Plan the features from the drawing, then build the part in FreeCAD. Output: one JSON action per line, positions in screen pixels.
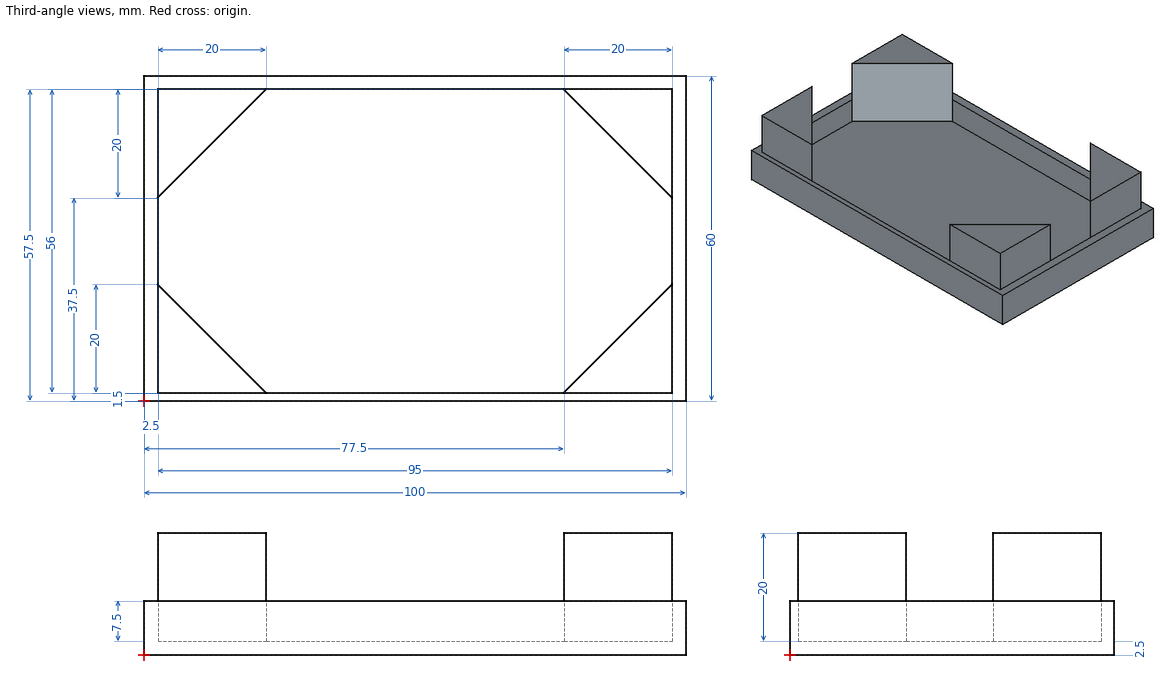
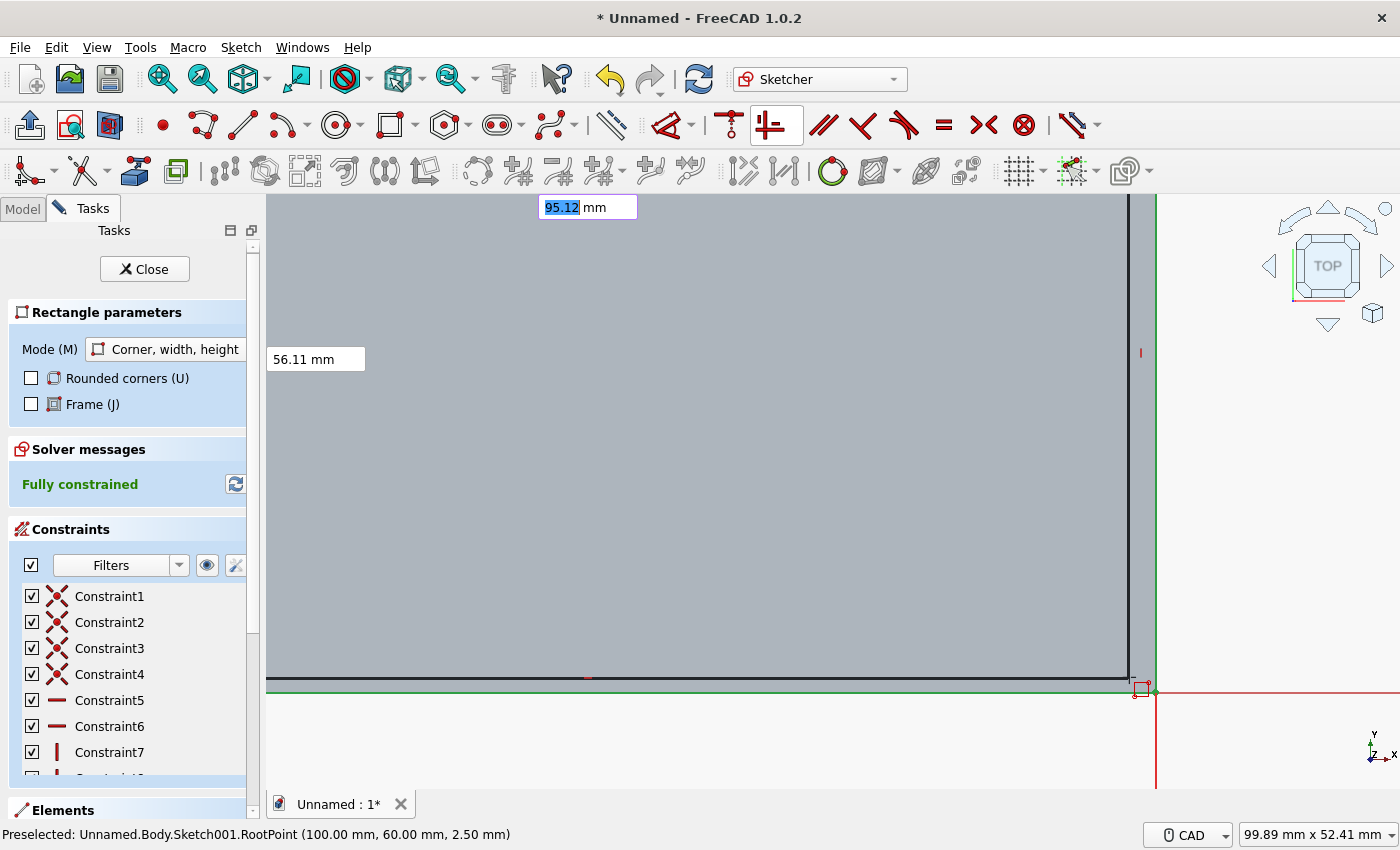
{"action": "left_click", "coordinate": [1128, 676]}
{"action": "key", "text": "Escape"}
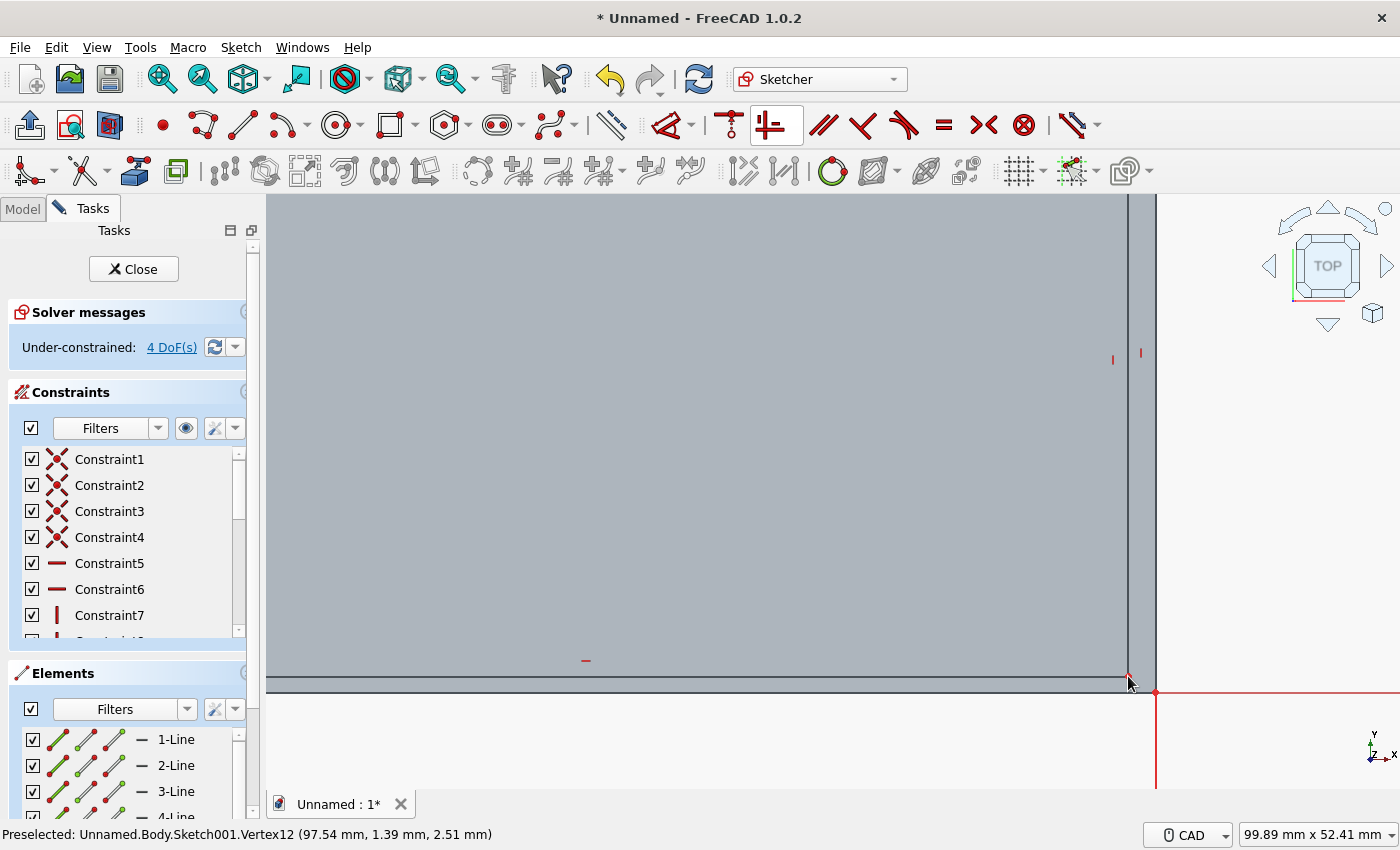
{"action": "left_click", "coordinate": [666, 126]}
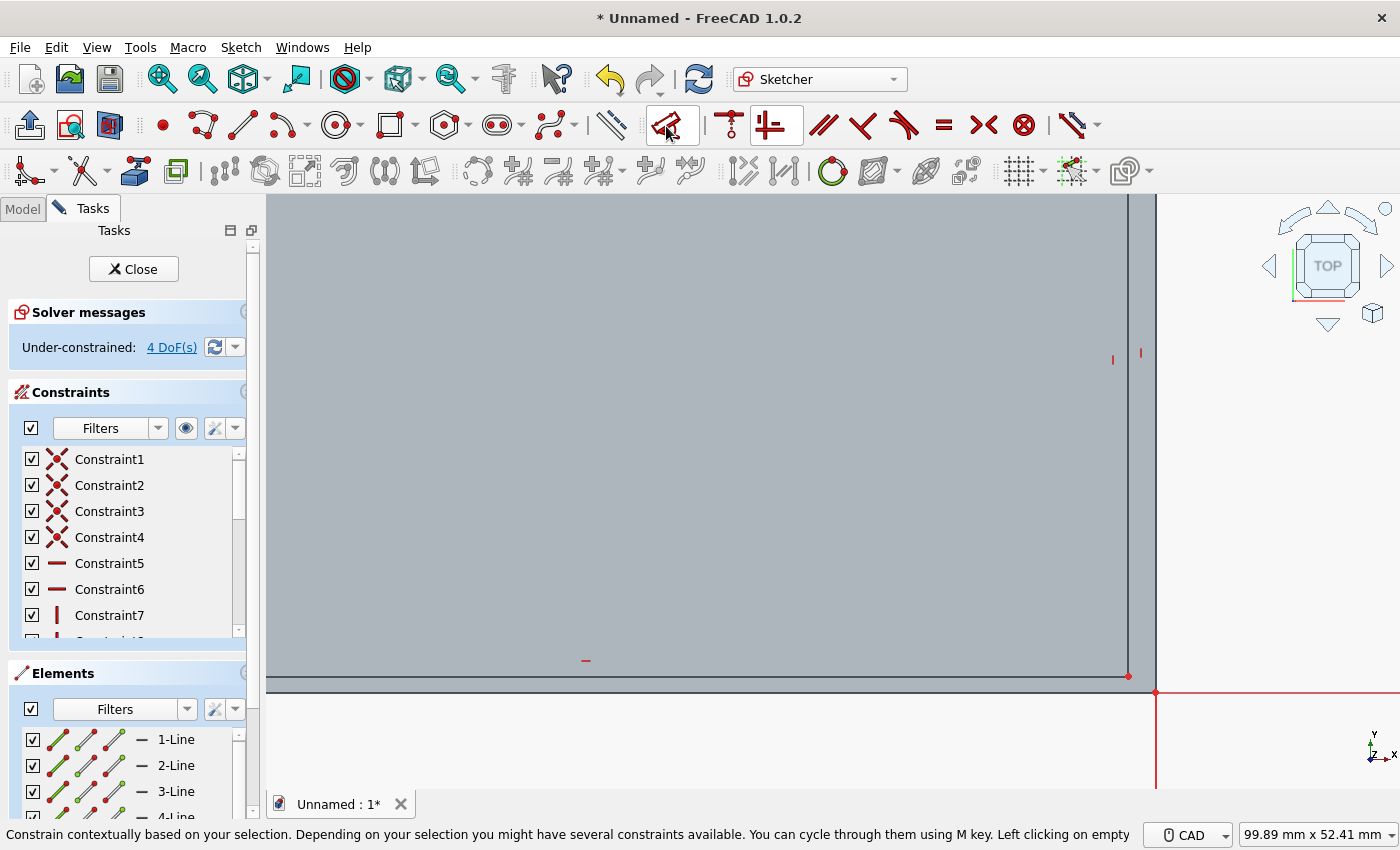
{"action": "scroll", "coordinate": [979, 661], "scroll_direction": "down", "scroll_amount": 3}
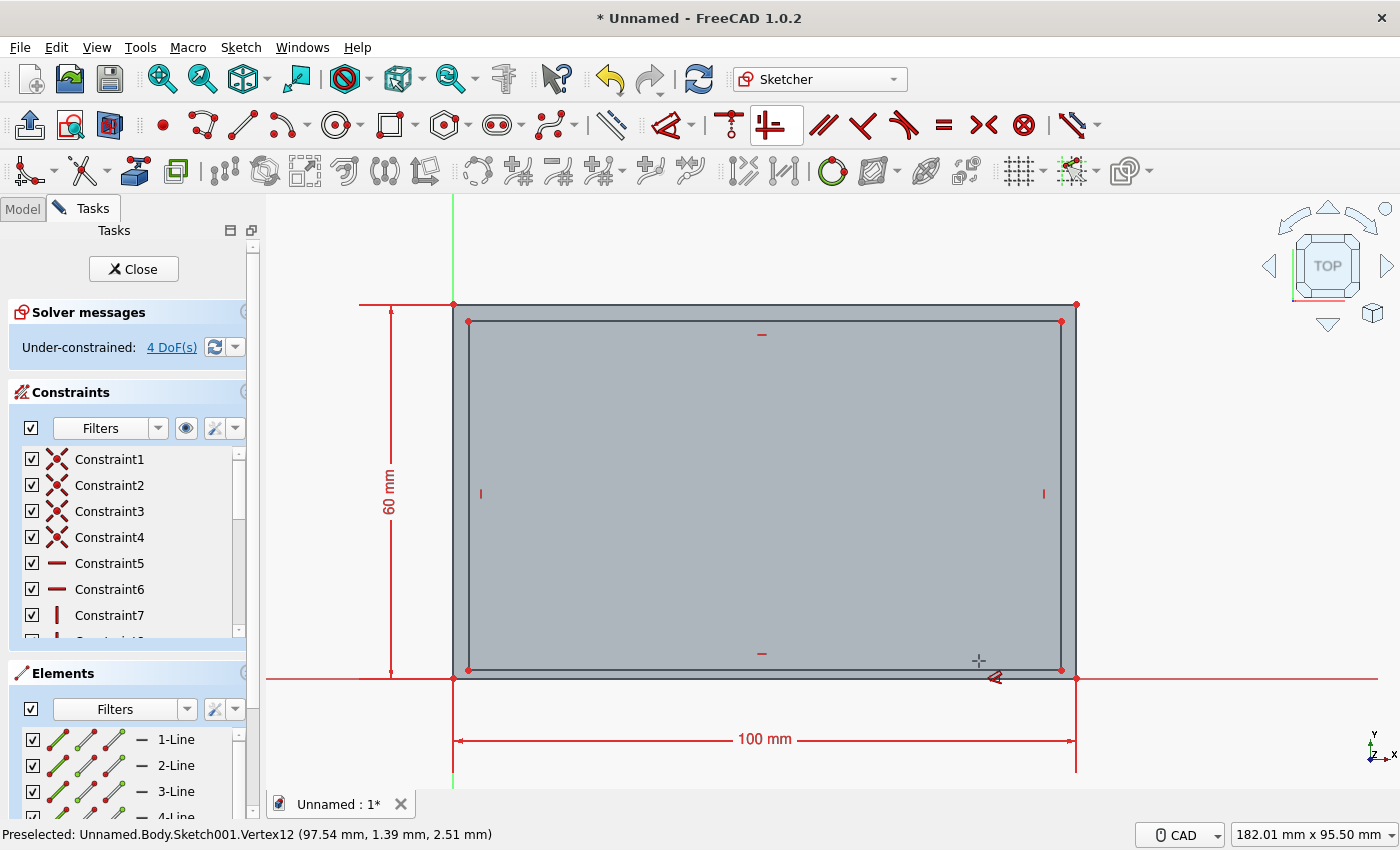
{"action": "left_click", "coordinate": [469, 426]}
{"action": "left_click", "coordinate": [435, 496]}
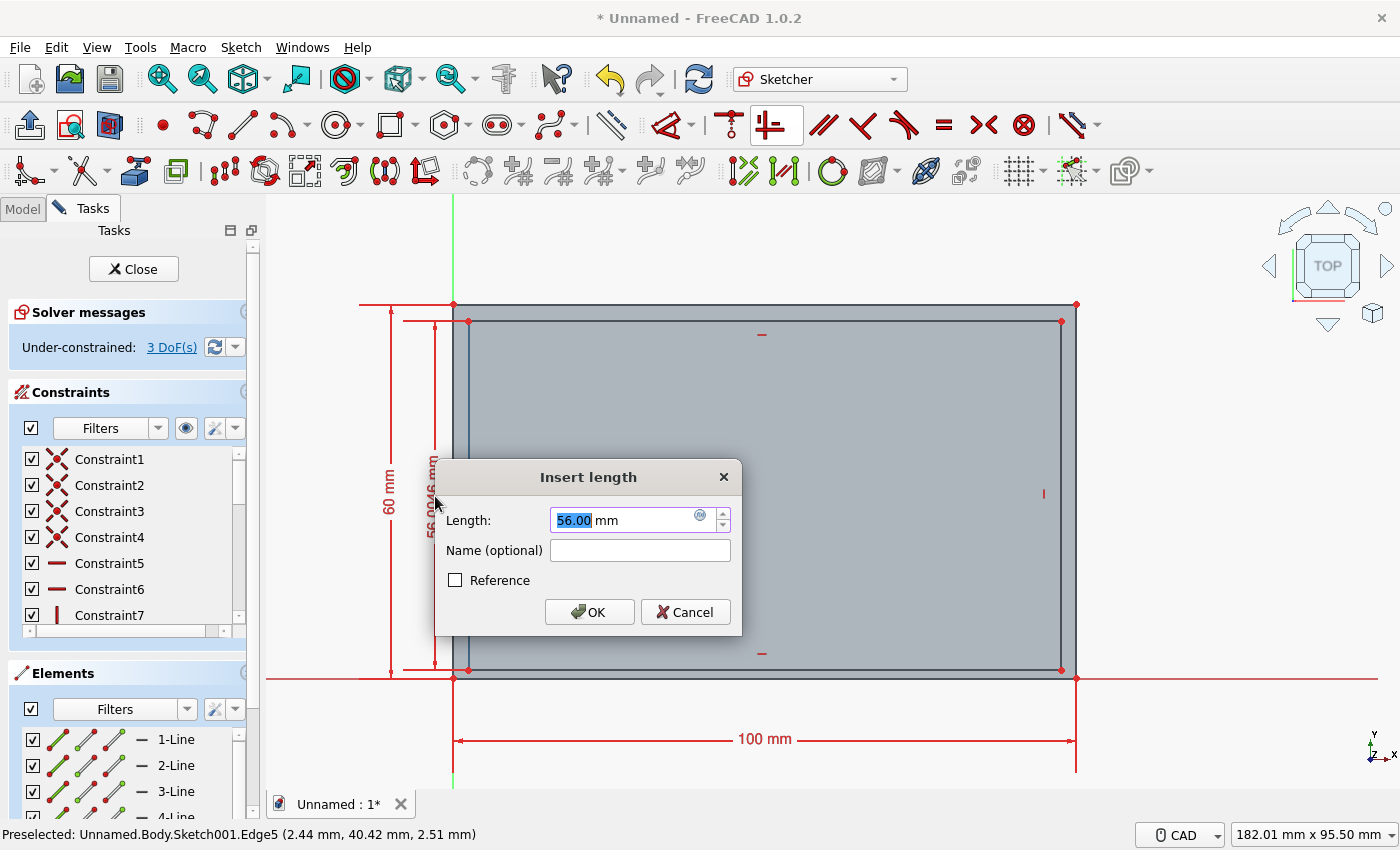
{"action": "type", "text": "56"}
{"action": "key", "text": "Return"}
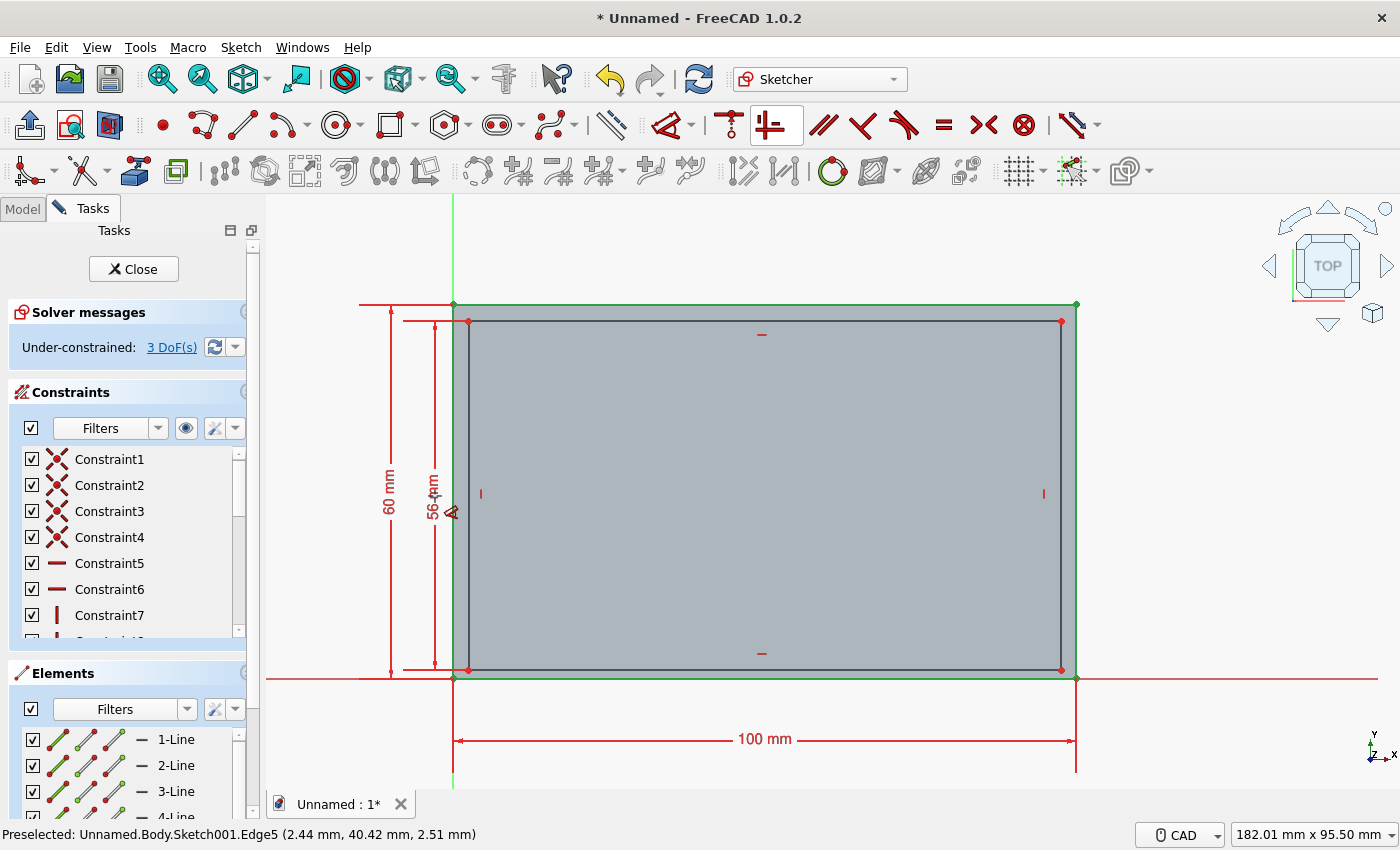
{"action": "scroll", "coordinate": [646, 670], "scroll_direction": "up", "scroll_amount": 3}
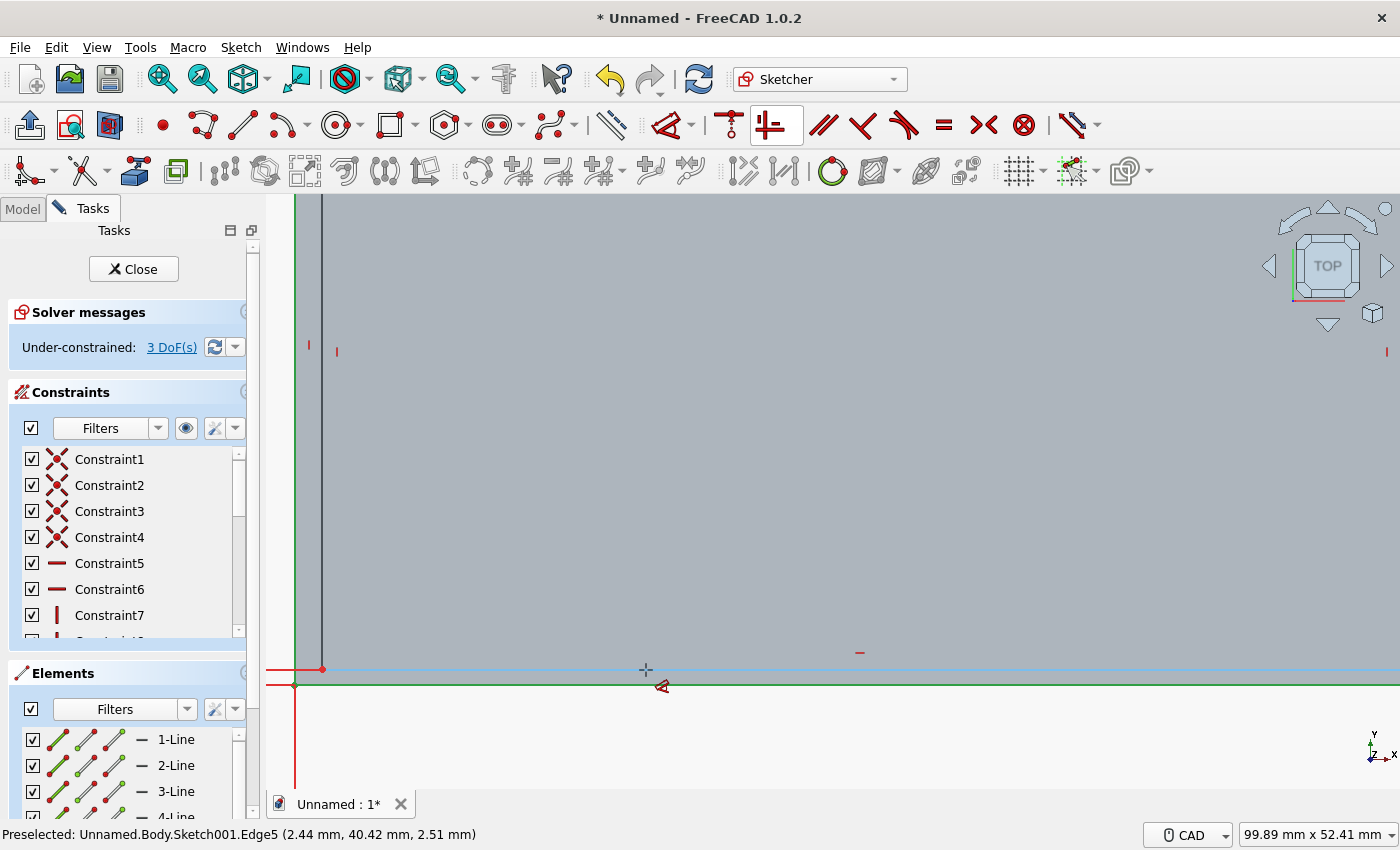
{"action": "left_click", "coordinate": [646, 670]}
{"action": "left_click", "coordinate": [779, 704]}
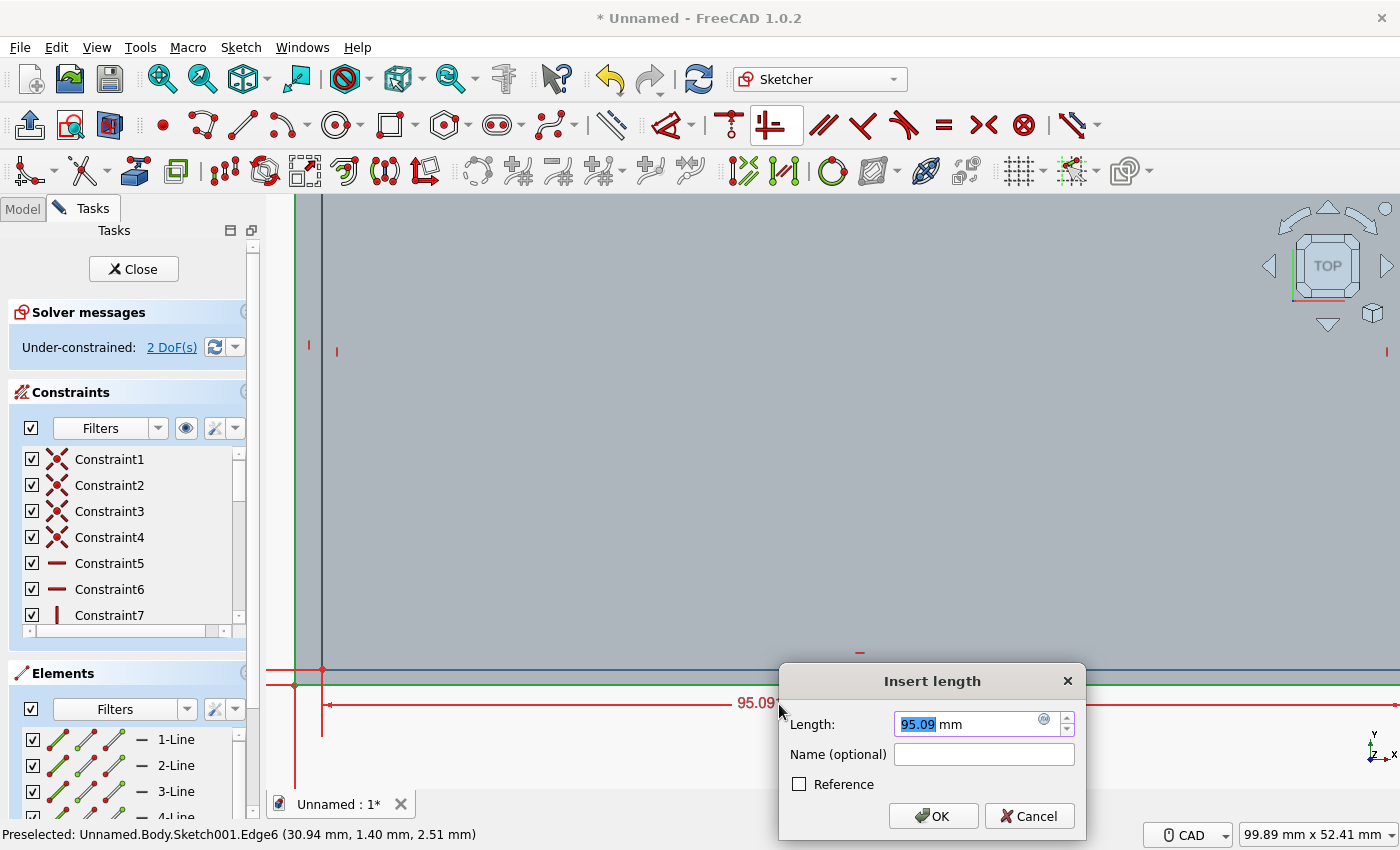
{"action": "type", "text": "95"}
{"action": "key", "text": "Return"}